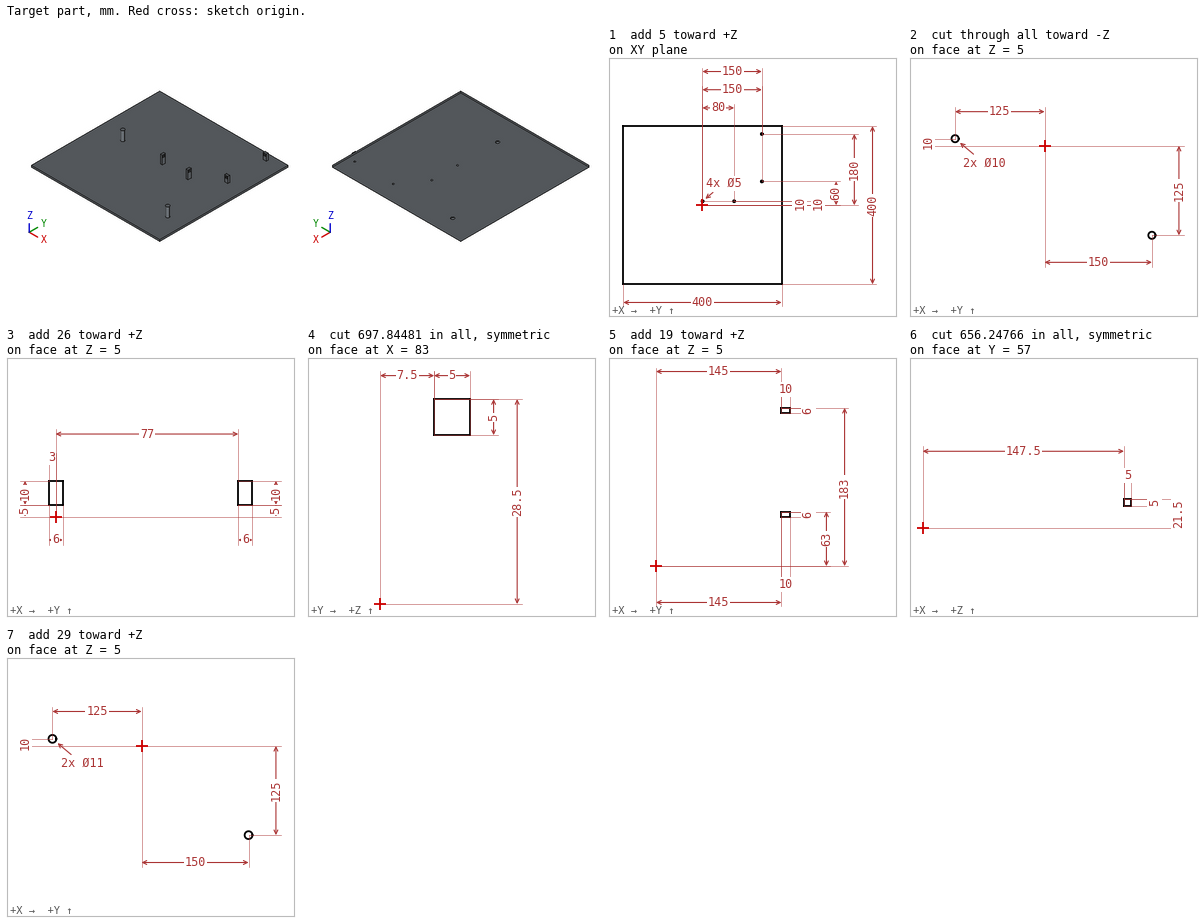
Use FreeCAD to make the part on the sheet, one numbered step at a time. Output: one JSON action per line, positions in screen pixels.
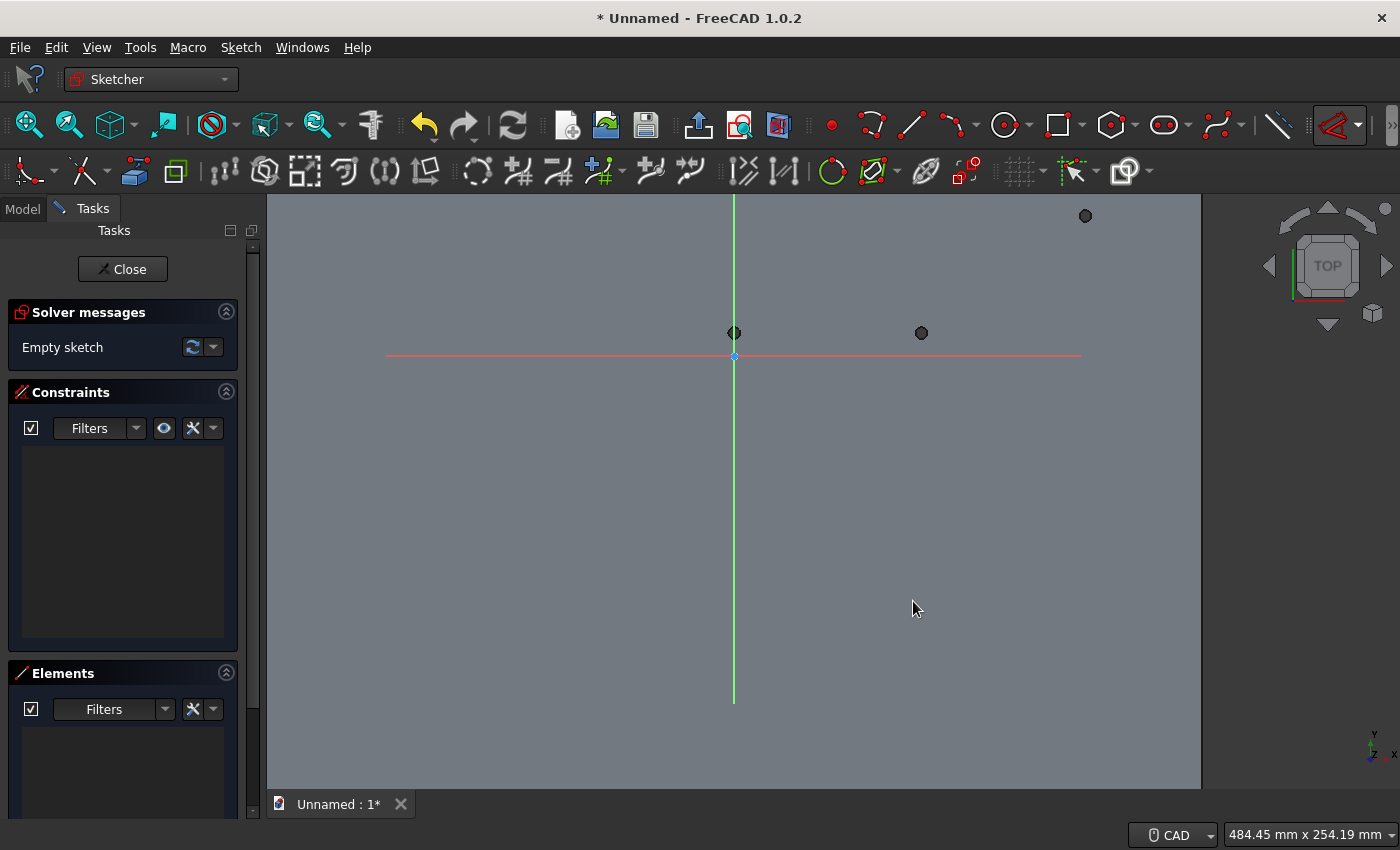
{"action": "key", "text": "g c"}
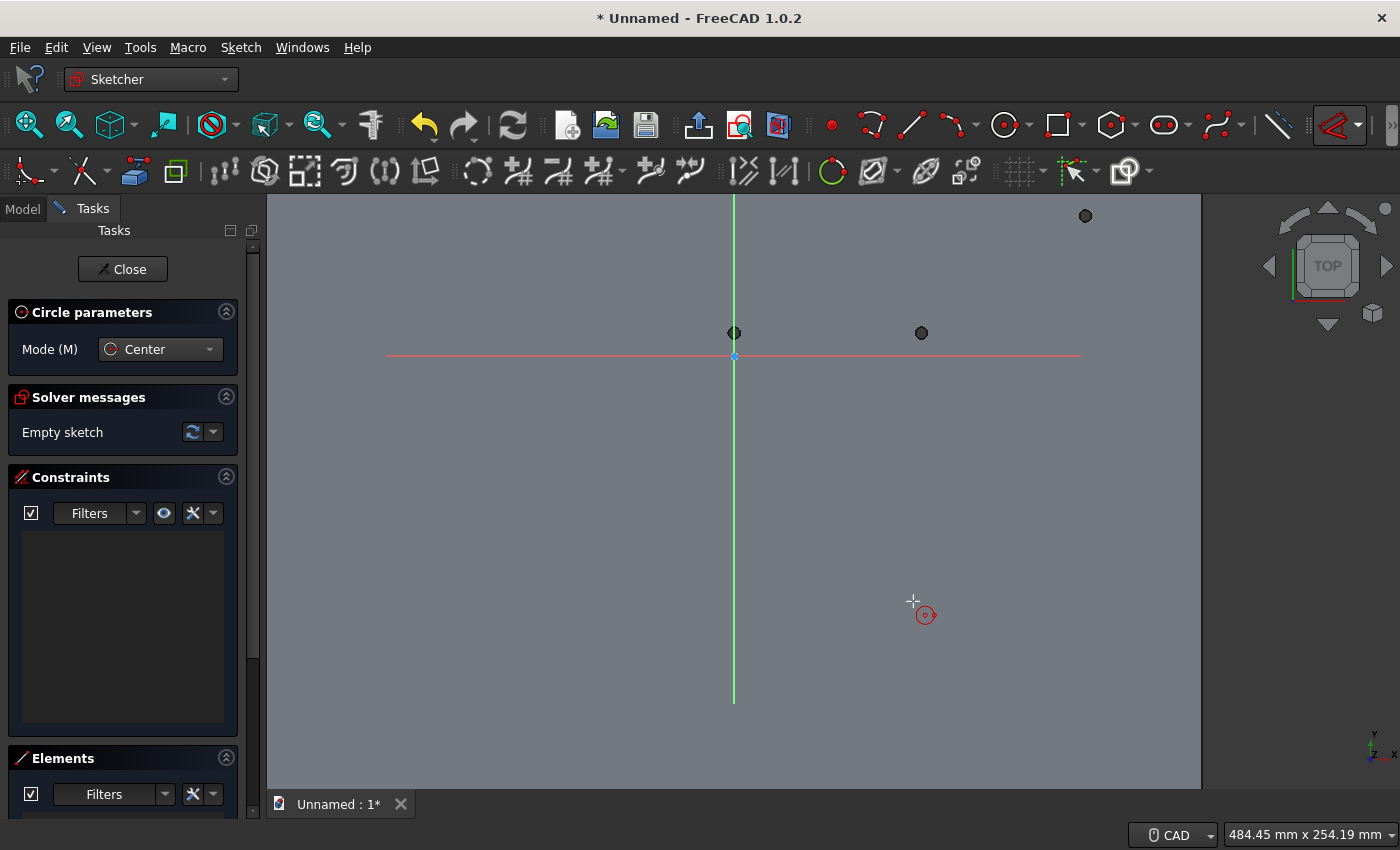
{"action": "scroll", "coordinate": [442, 333], "scroll_direction": "up", "scroll_amount": 4}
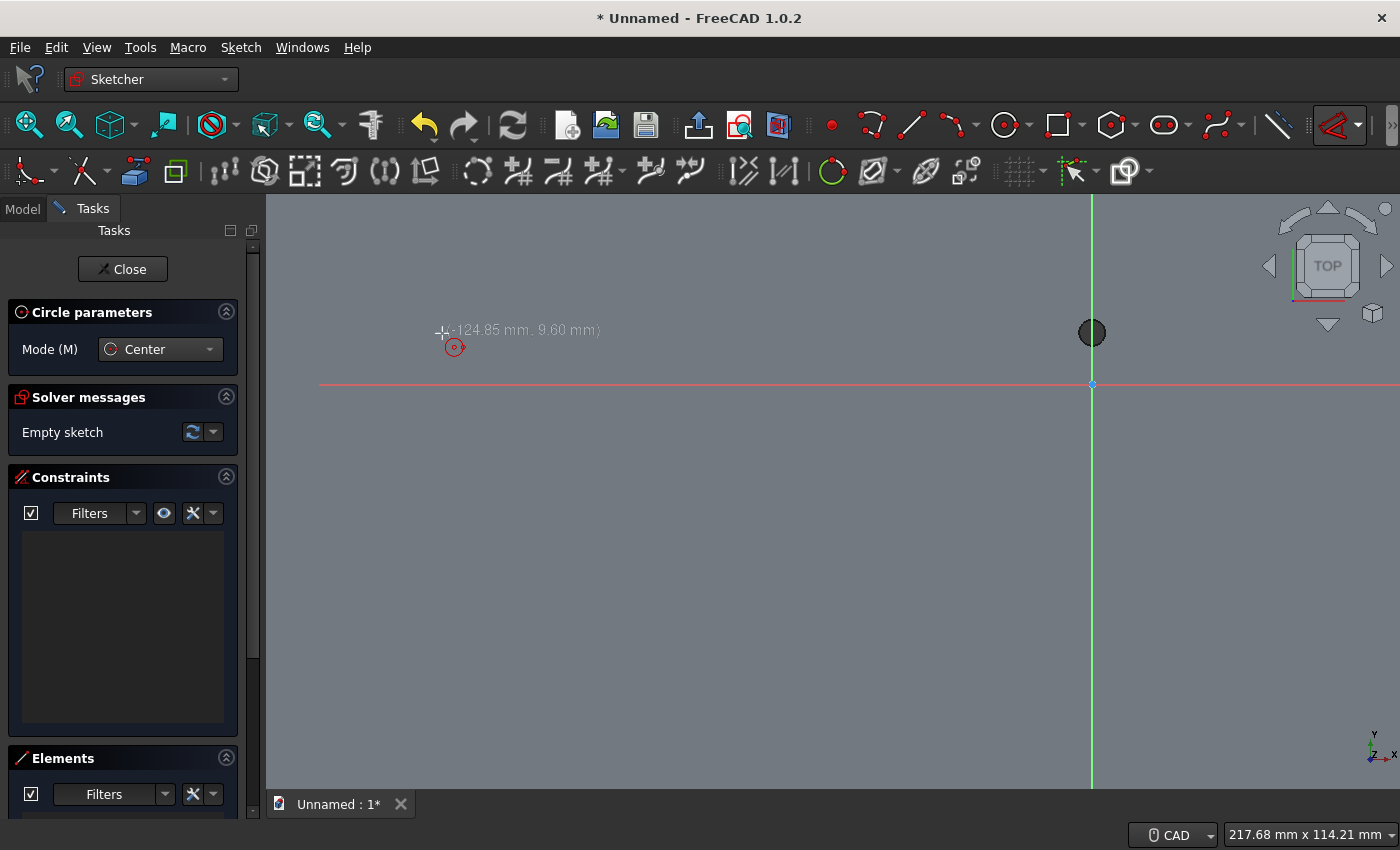
{"action": "left_click", "coordinate": [441, 333]}
{"action": "left_click", "coordinate": [459, 314]}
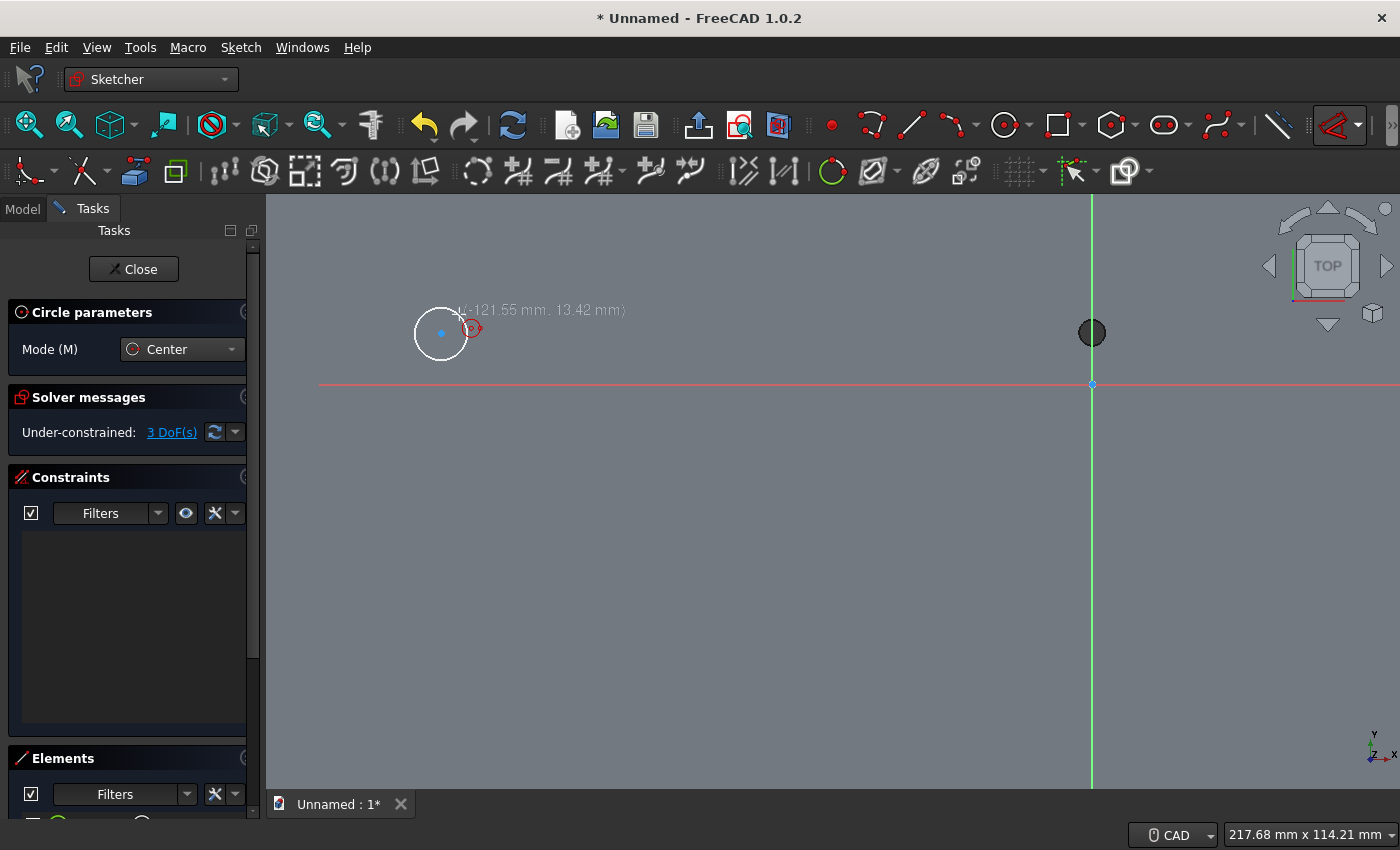
{"action": "scroll", "coordinate": [444, 334], "scroll_direction": "down", "scroll_amount": 4}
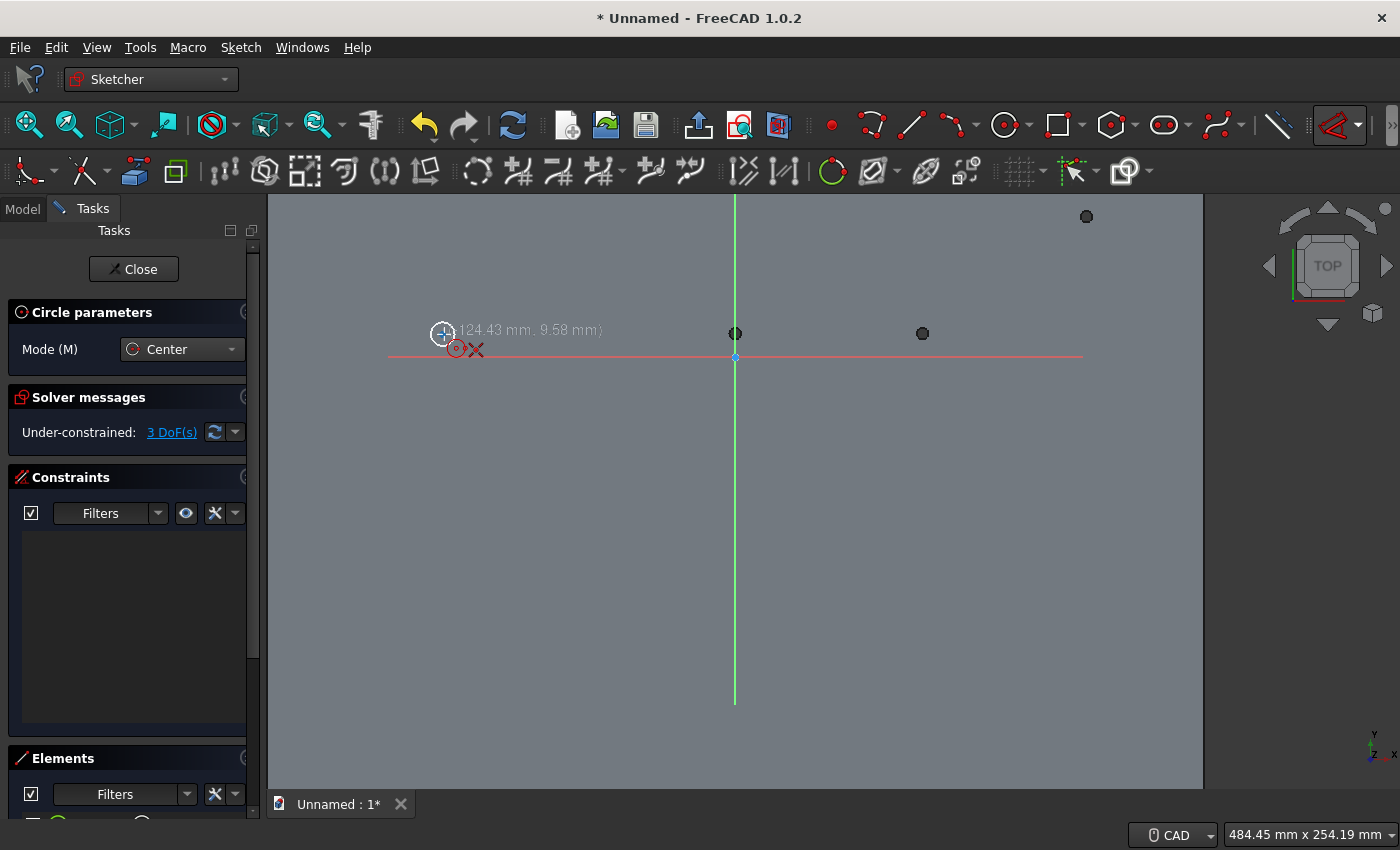
{"action": "scroll", "coordinate": [1086, 650], "scroll_direction": "up", "scroll_amount": 4}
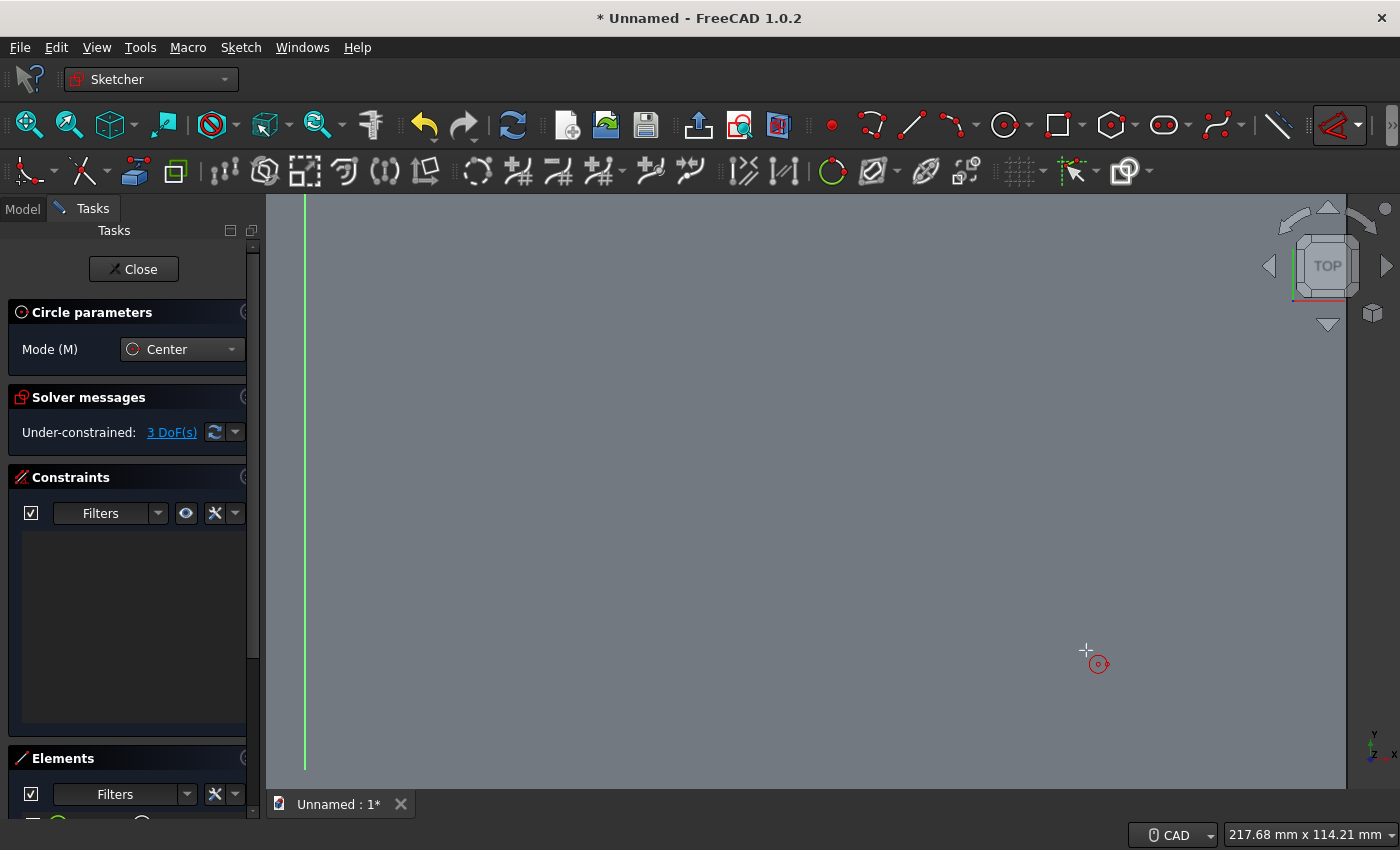
{"action": "left_click", "coordinate": [1086, 648]}
{"action": "left_click", "coordinate": [1105, 630]}
{"action": "key", "text": "Escape"}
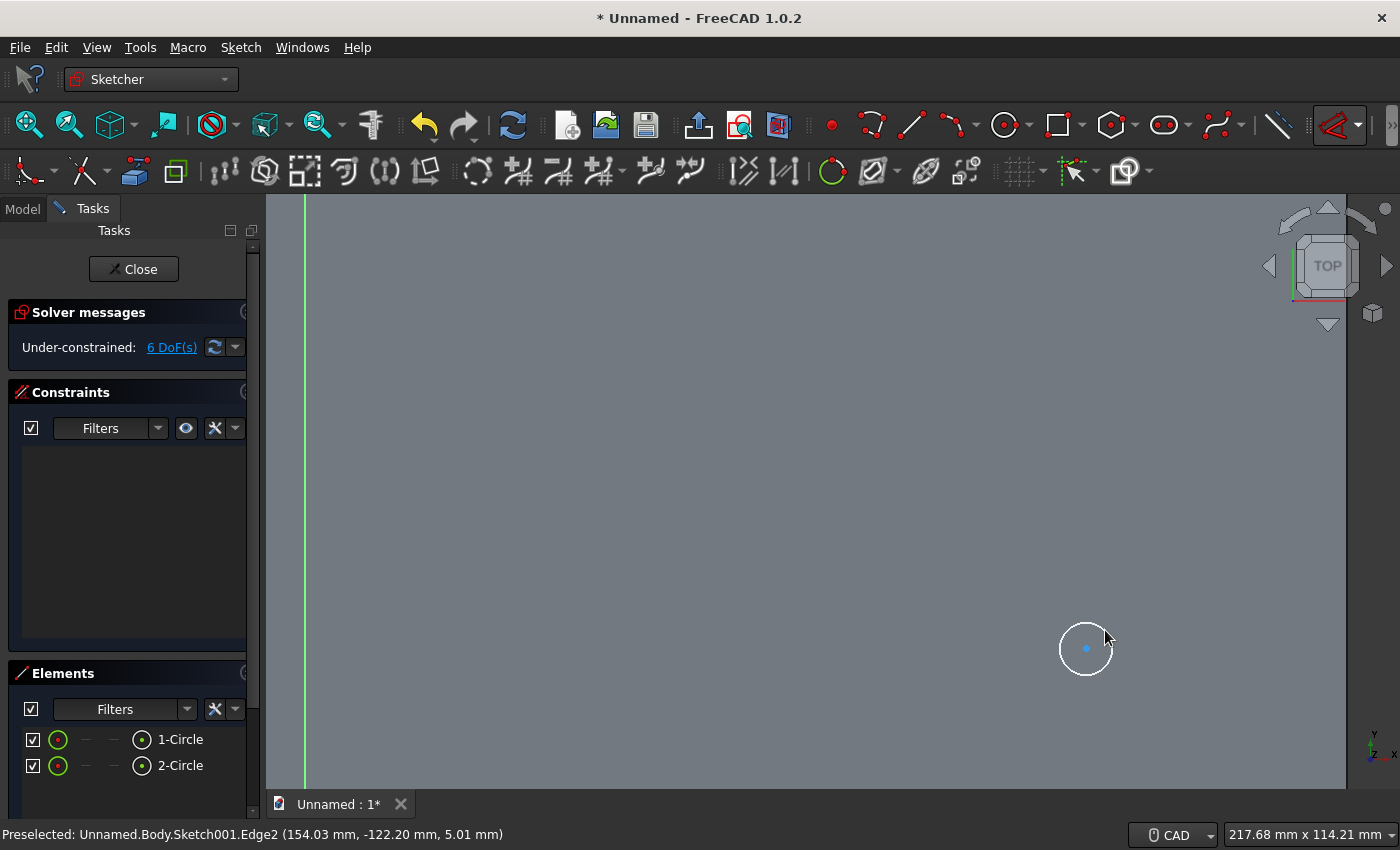
{"action": "scroll", "coordinate": [1087, 651], "scroll_direction": "down", "scroll_amount": 4}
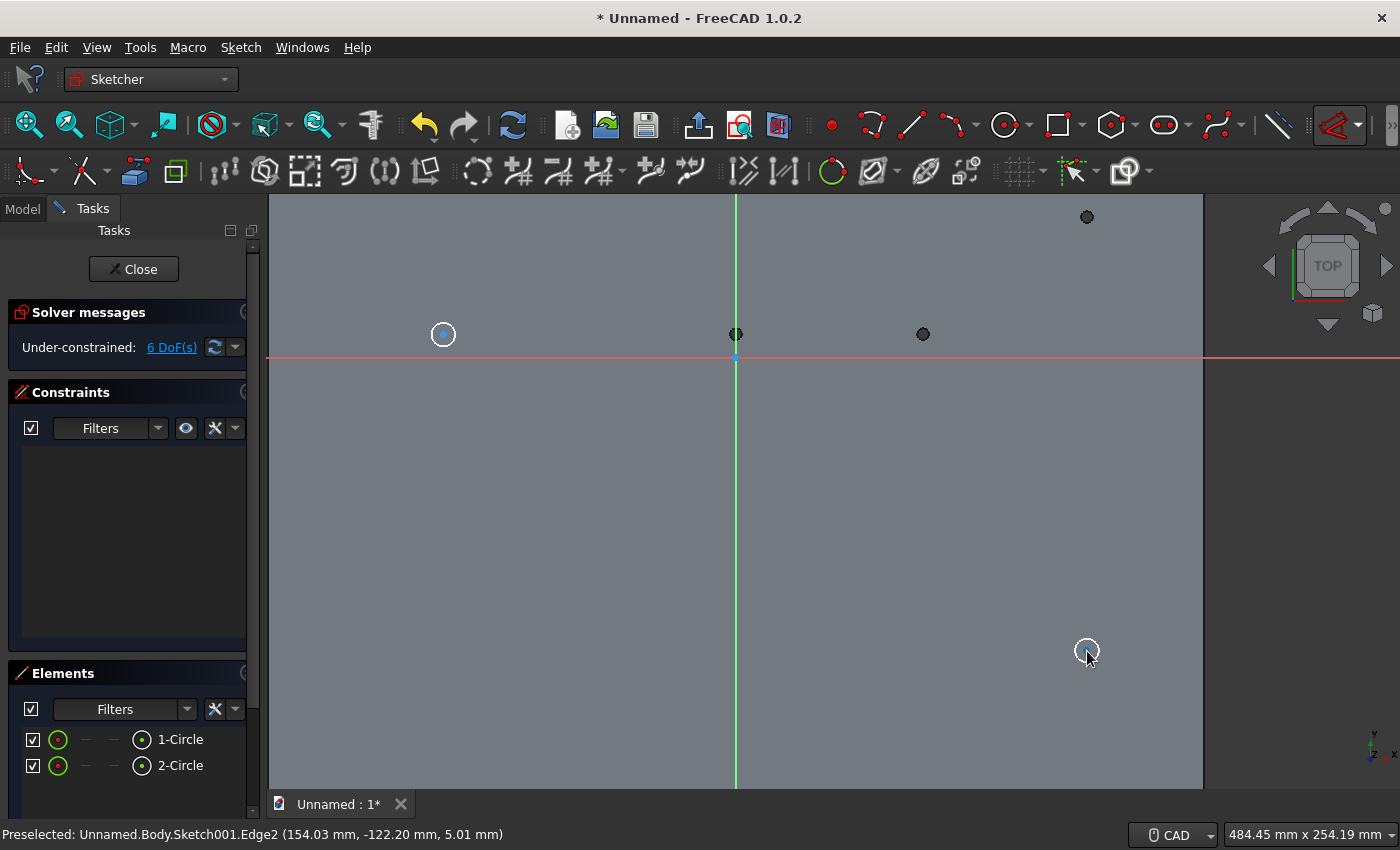
{"action": "left_click", "coordinate": [452, 326]}